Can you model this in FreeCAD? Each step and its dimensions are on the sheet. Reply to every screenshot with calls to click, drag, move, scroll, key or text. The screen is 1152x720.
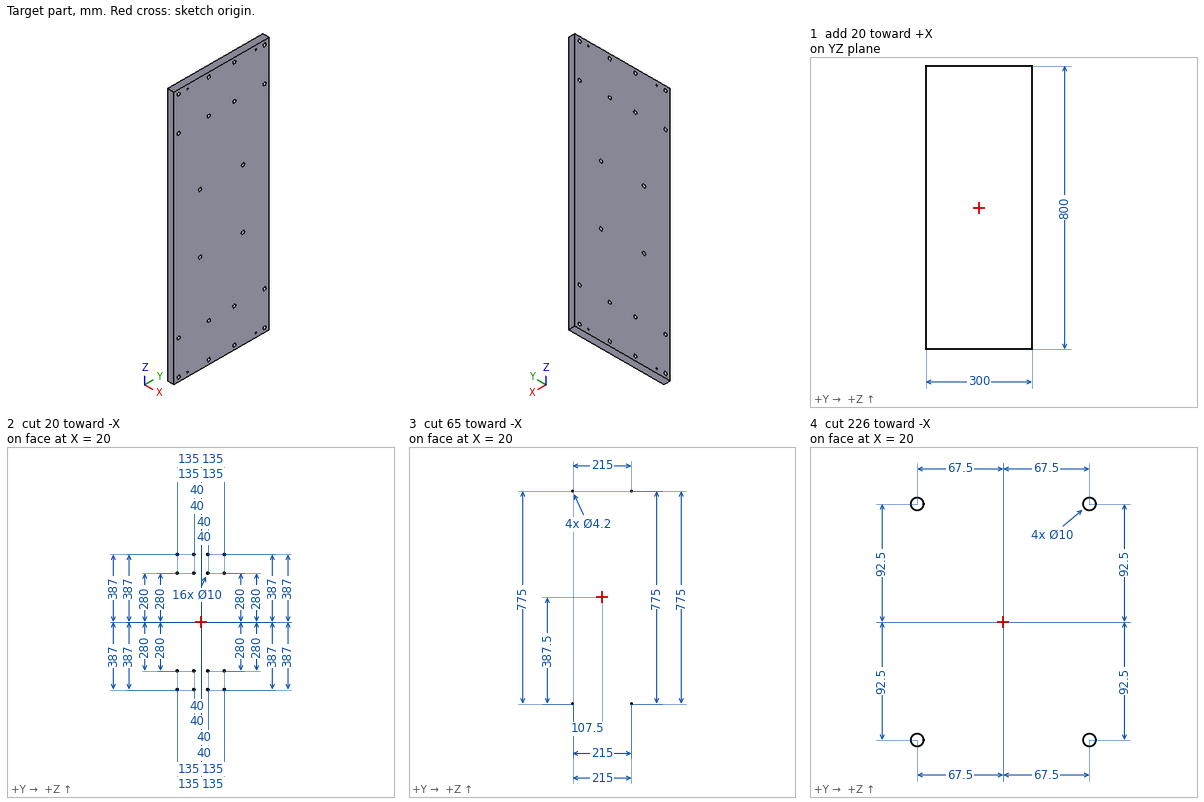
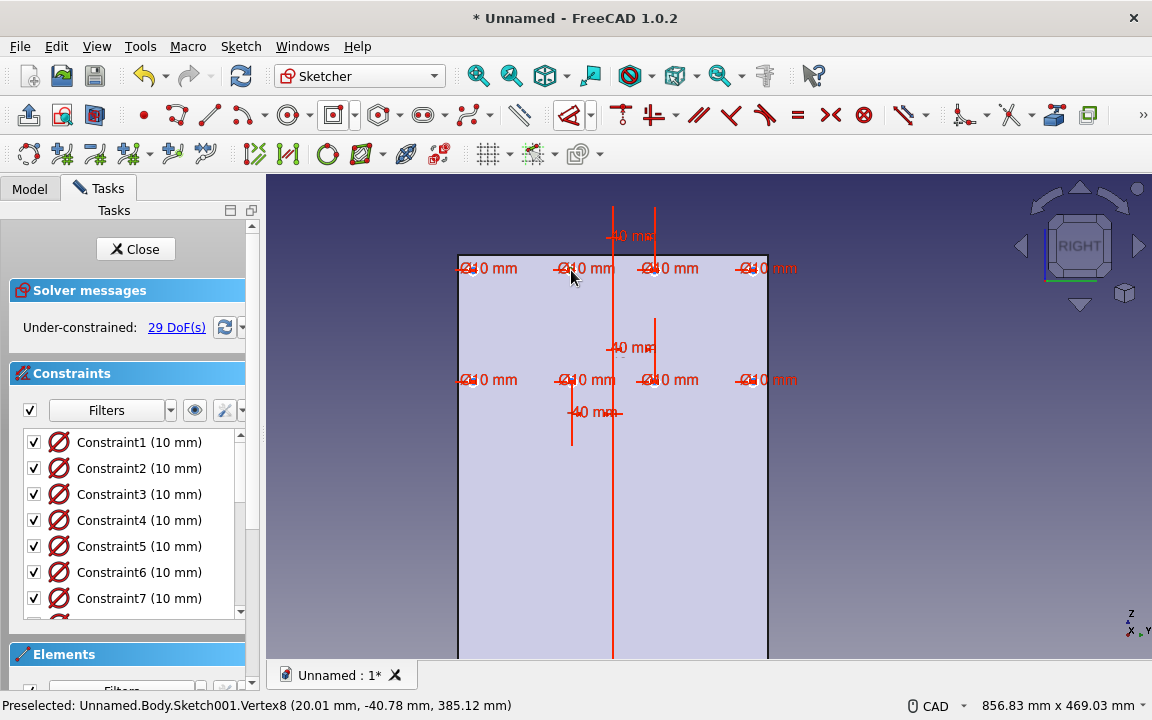
key(l)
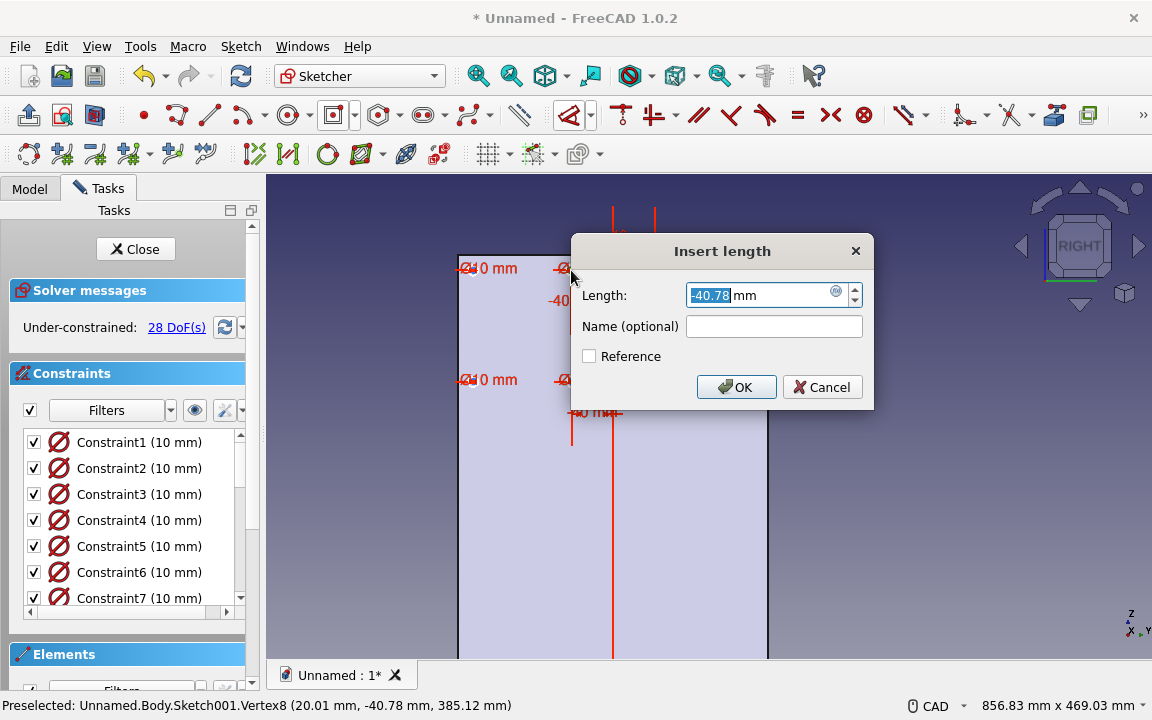
text(-40)
key(Return)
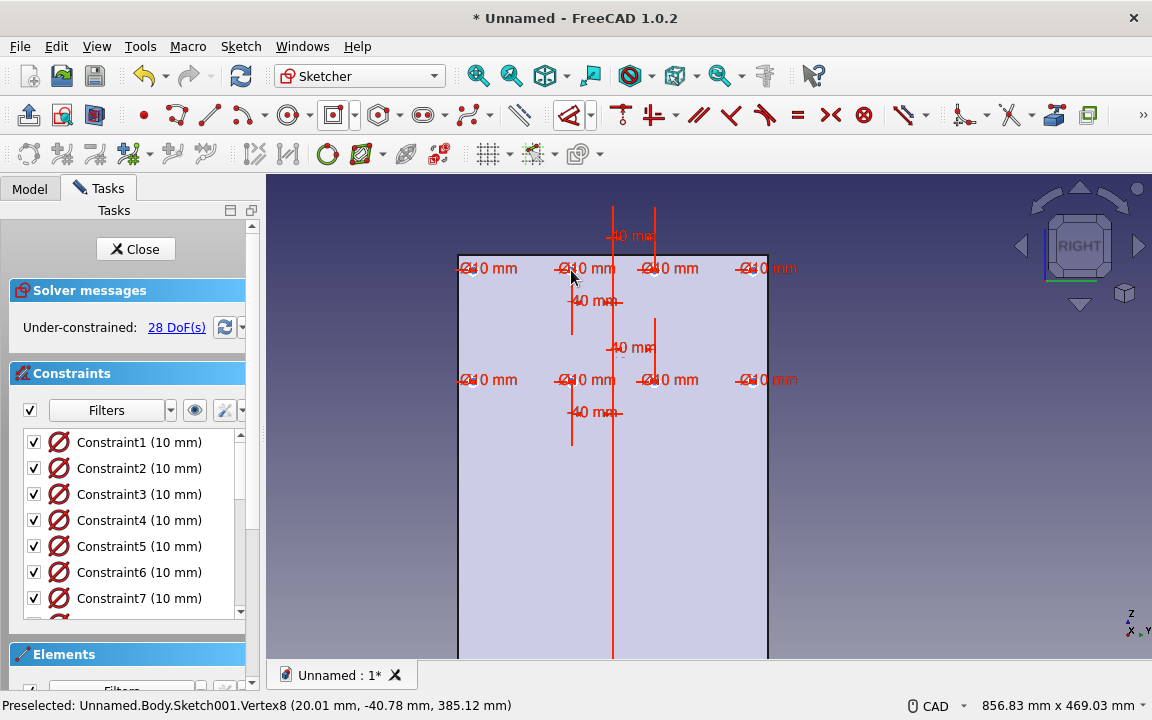
scroll(656, 270, down, 5)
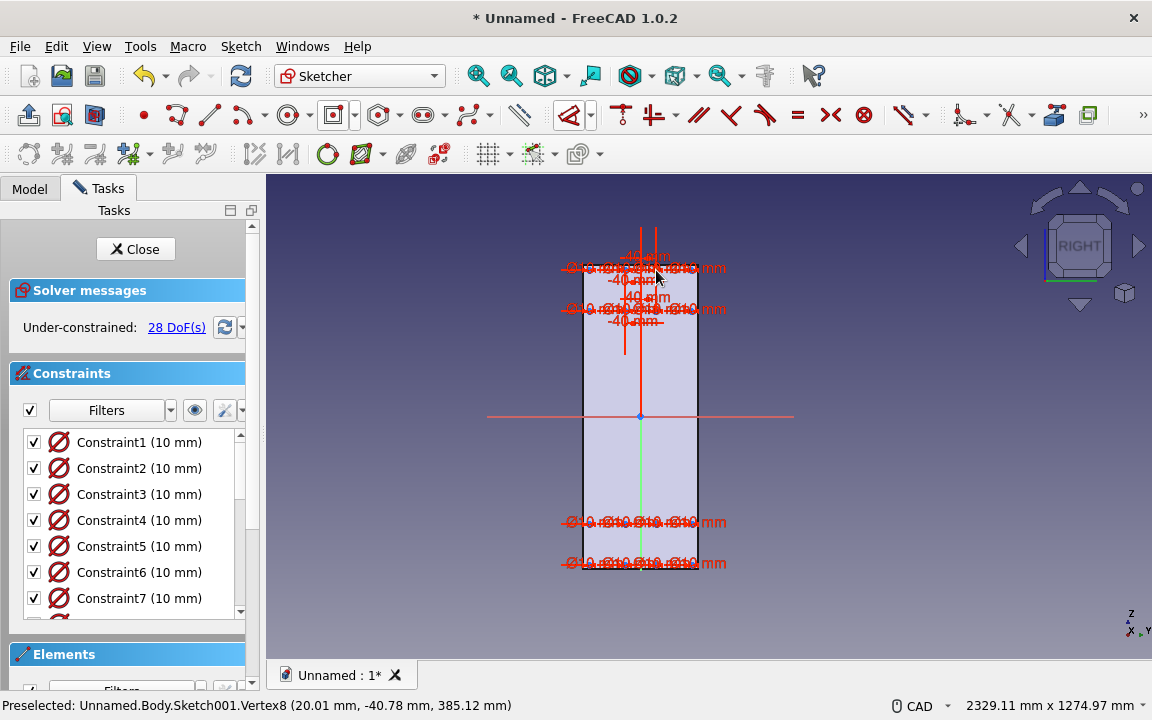
scroll(625, 524, up, 5)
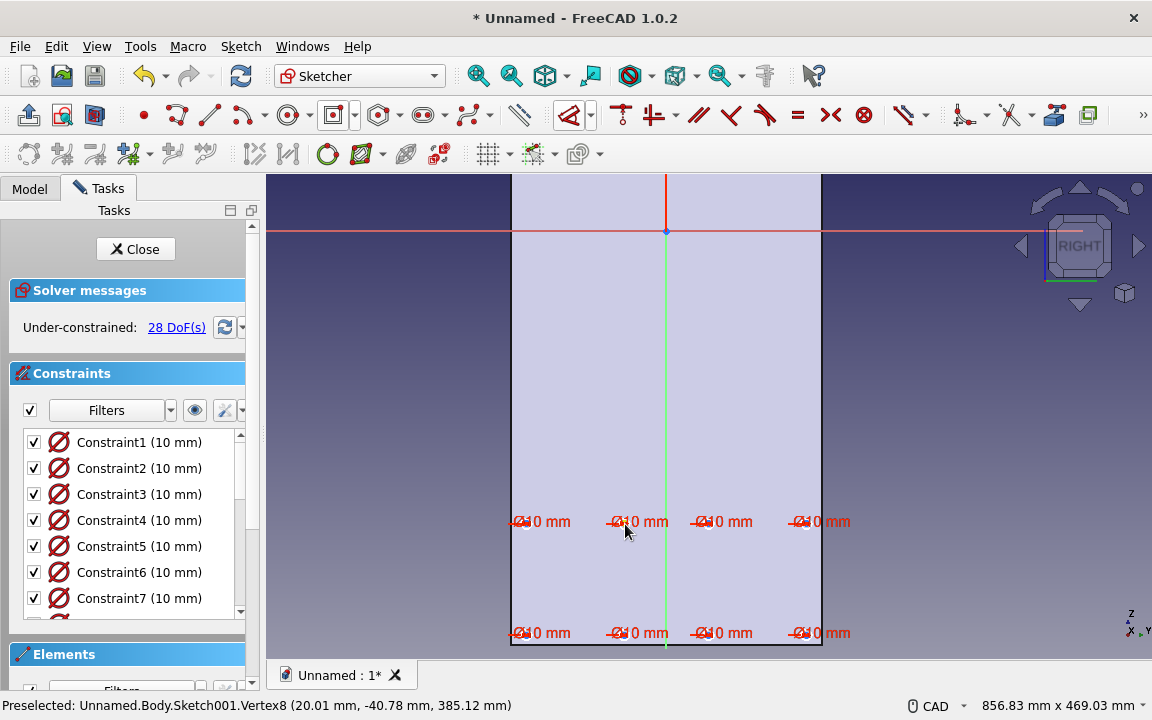
click(624, 524)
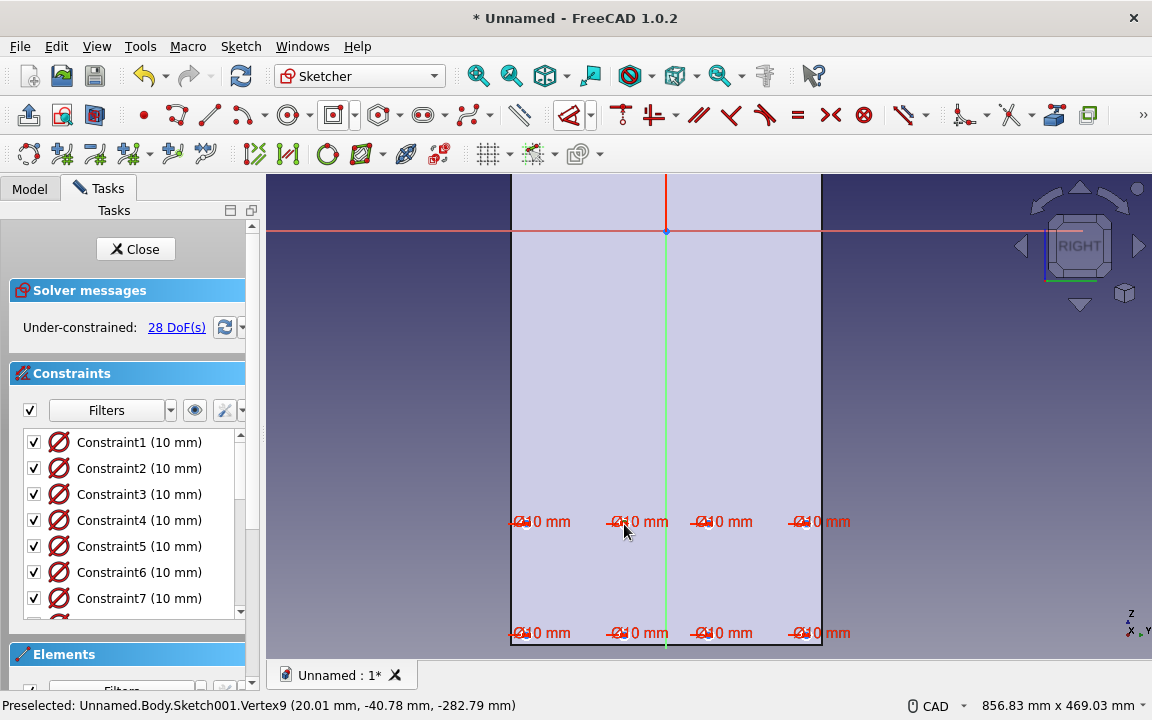
key(l)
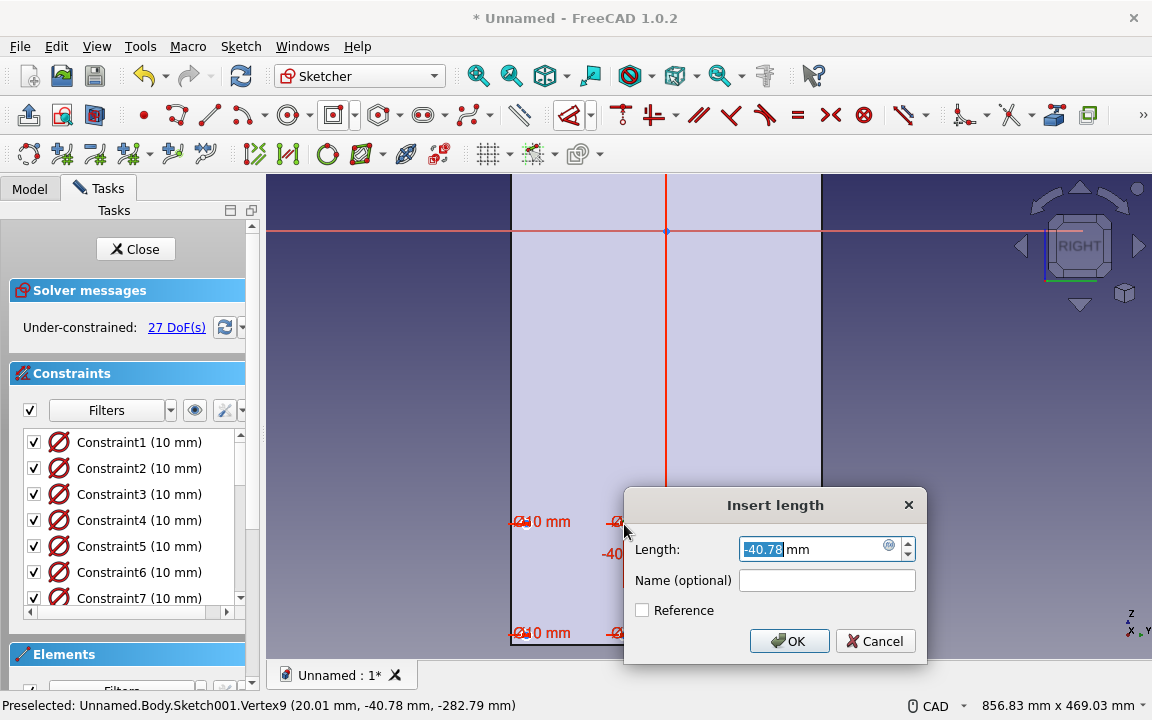
text(-40)
key(Return)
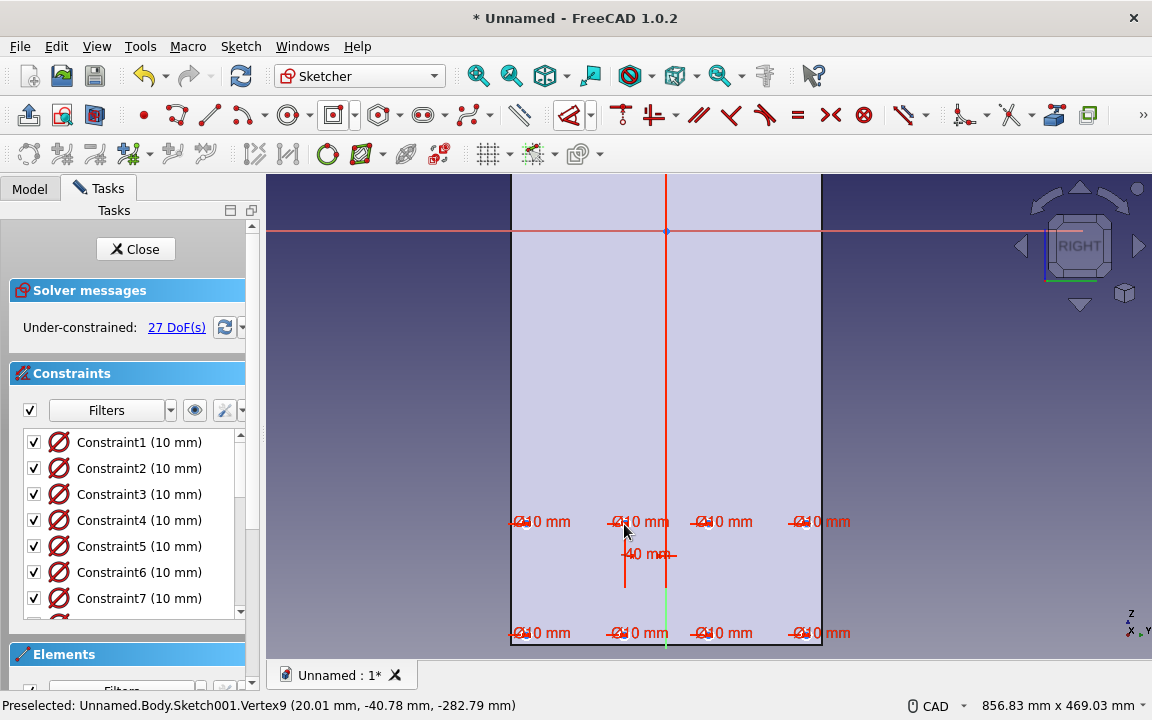
scroll(625, 524, down, 5)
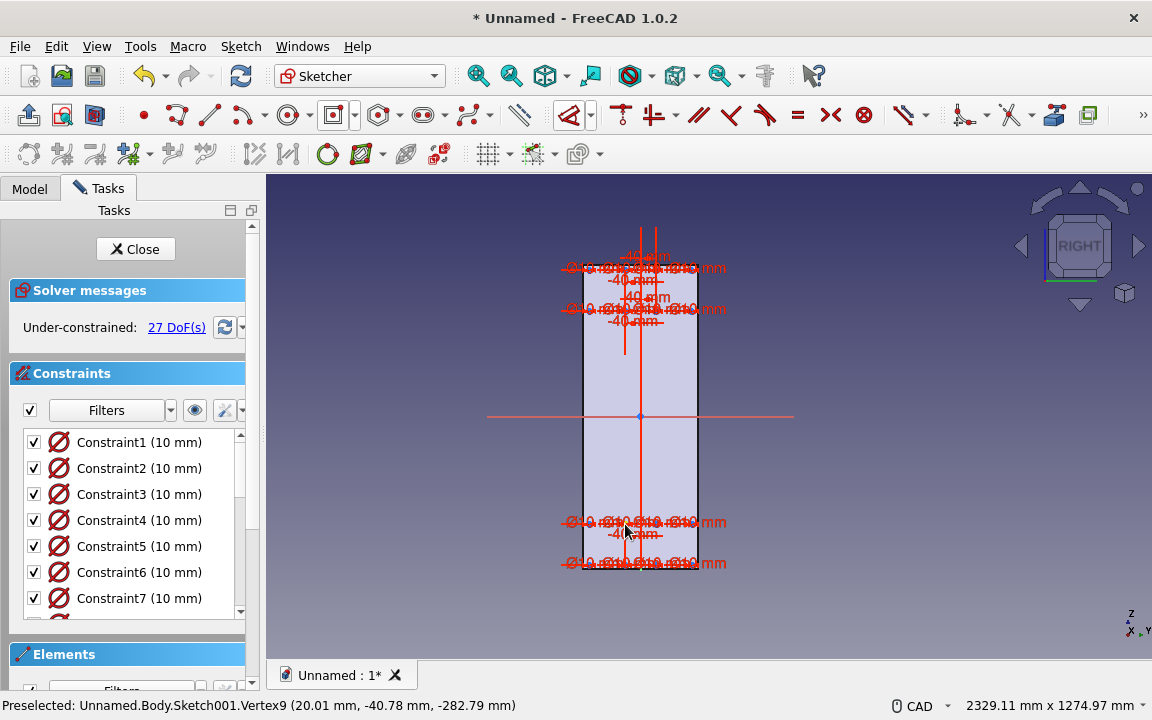
scroll(625, 565, up, 5)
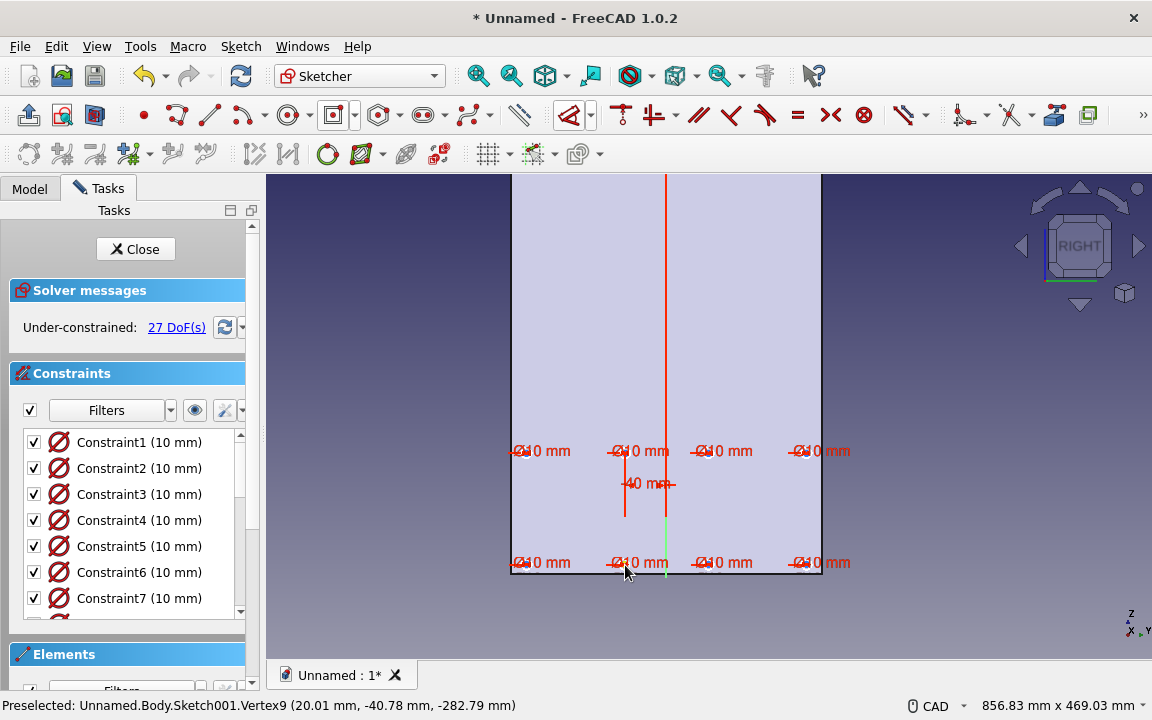
click(624, 565)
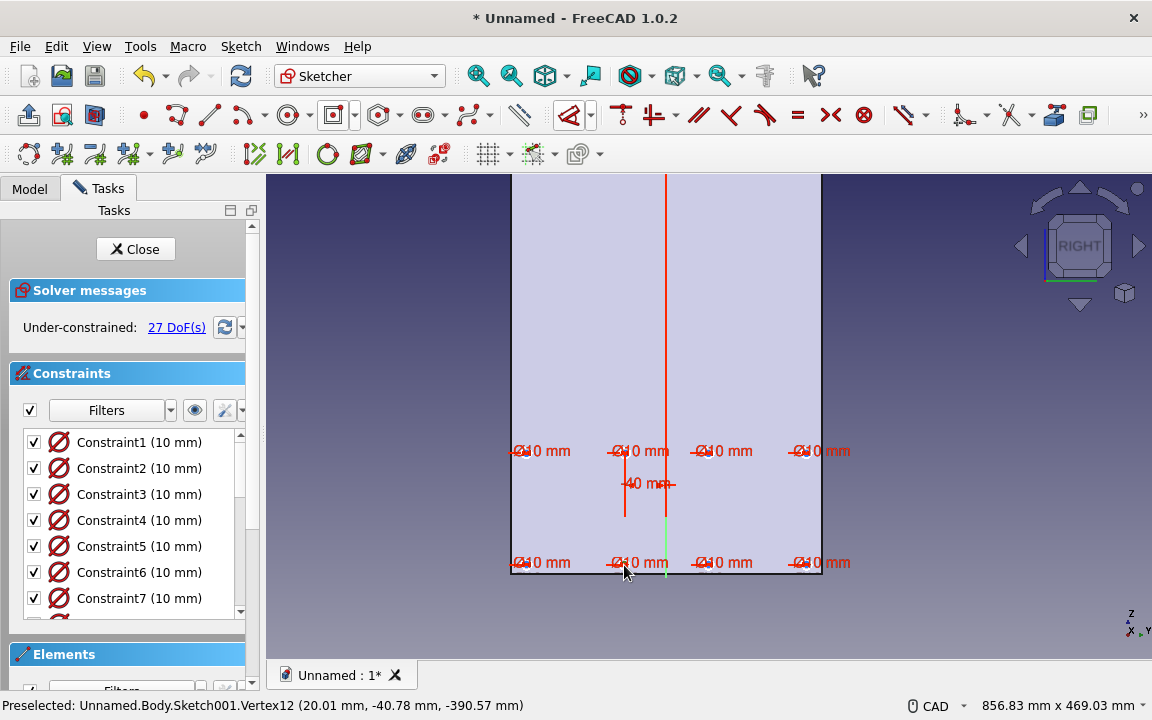
key(l)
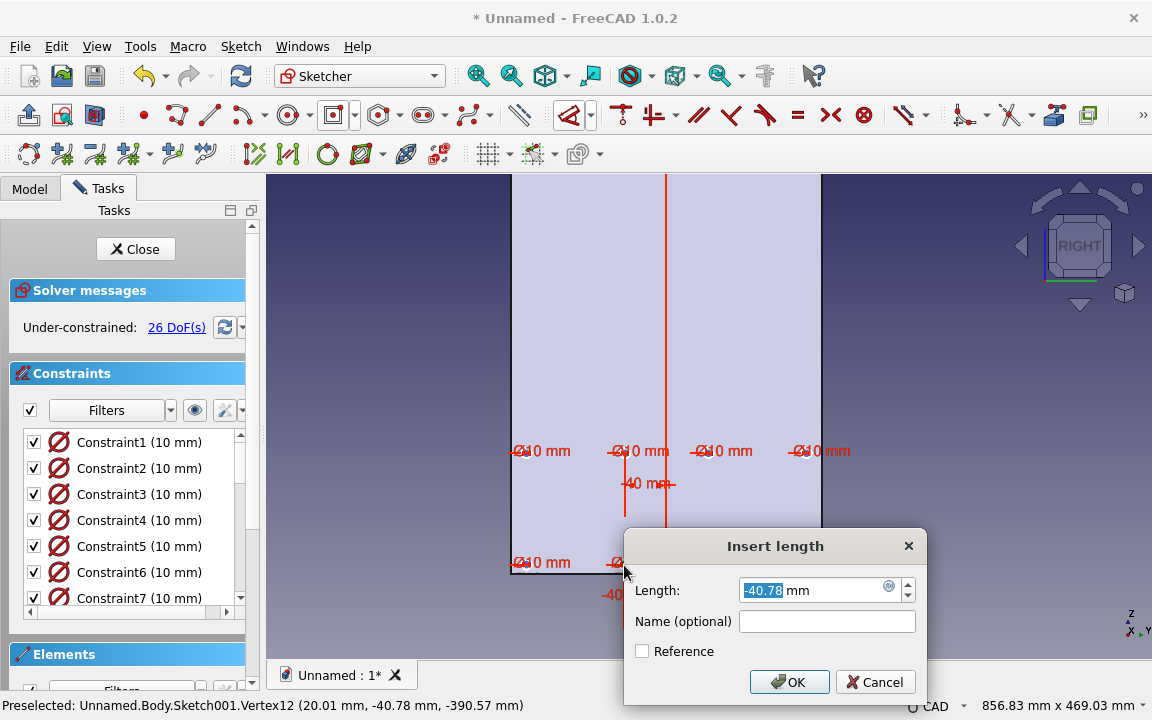
text(-40)
key(Return)